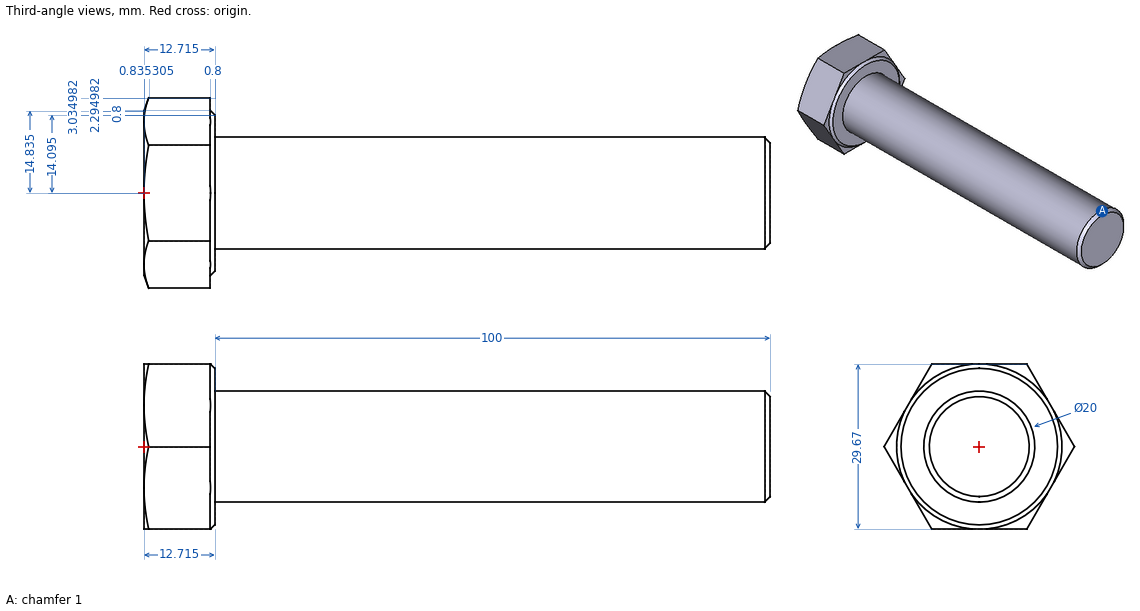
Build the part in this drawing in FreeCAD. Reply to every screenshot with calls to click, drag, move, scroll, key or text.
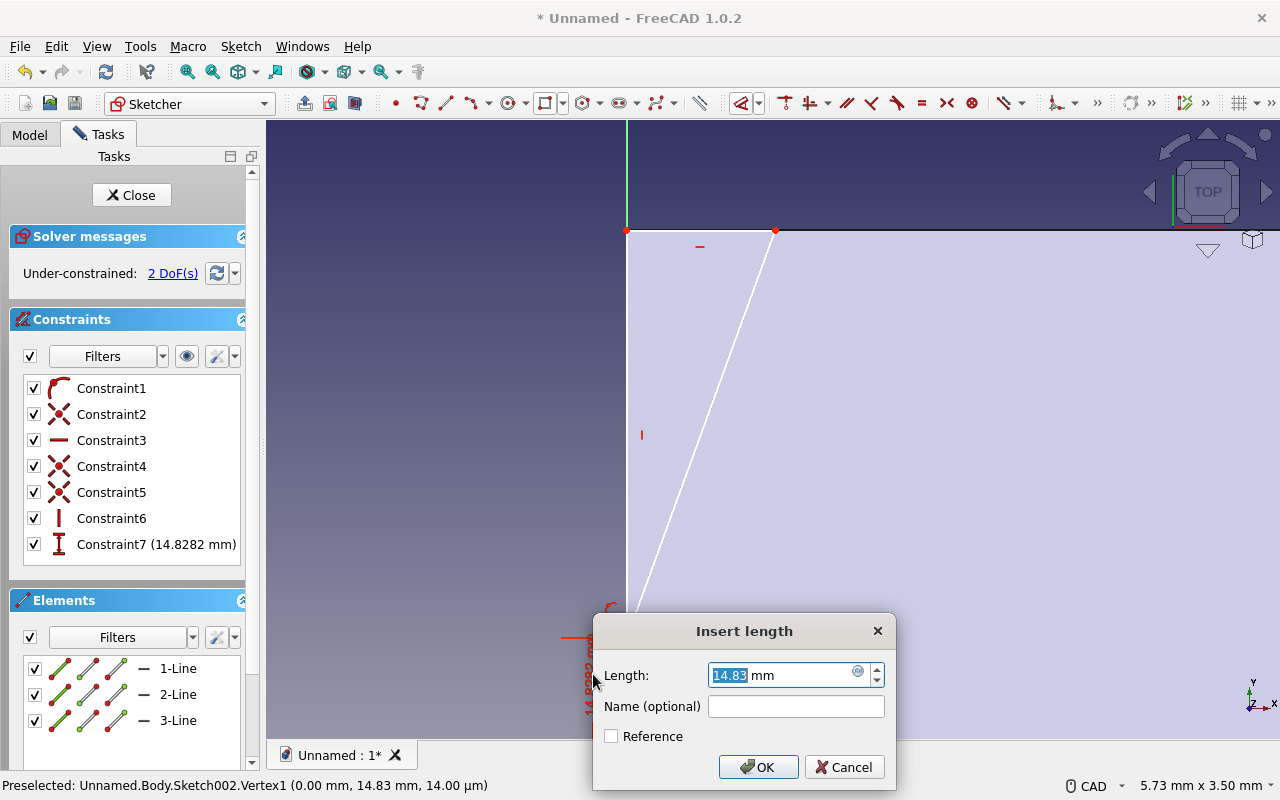
text(14.835)
key(Return)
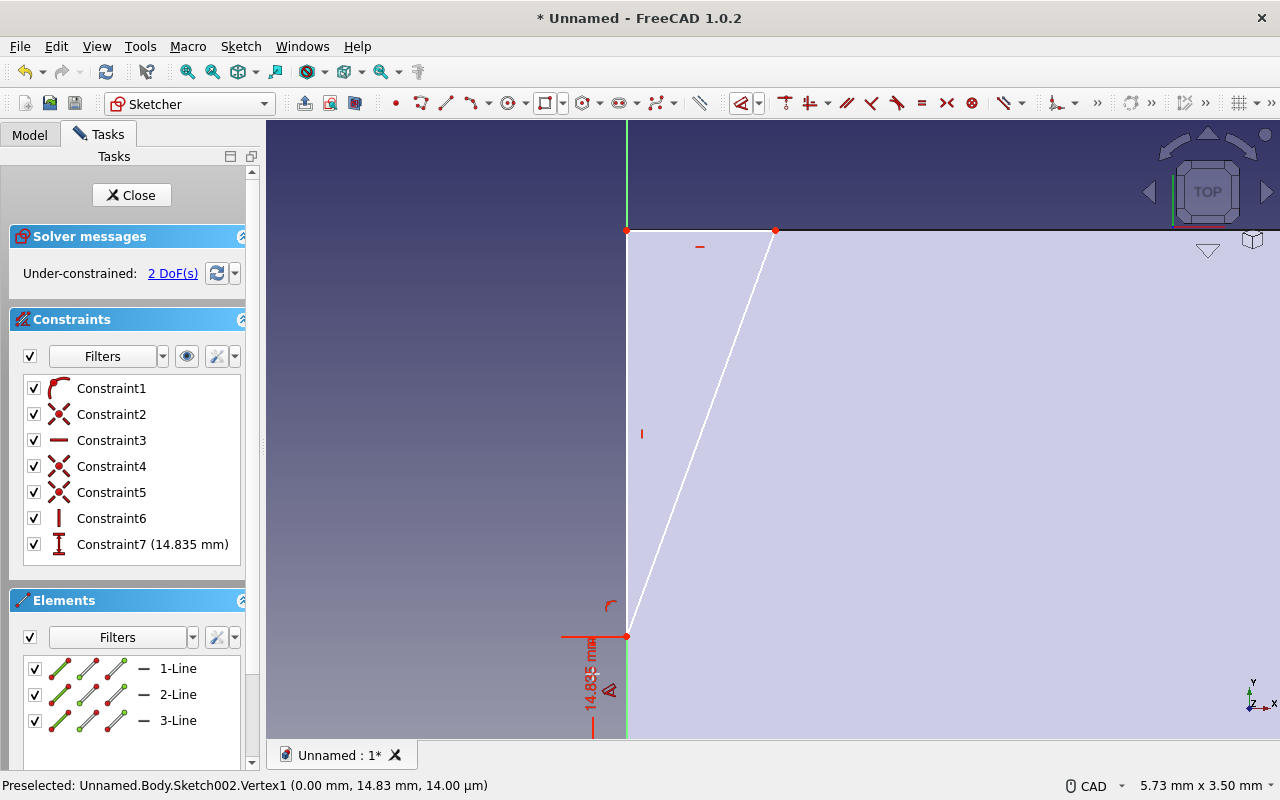
click(731, 231)
click(701, 197)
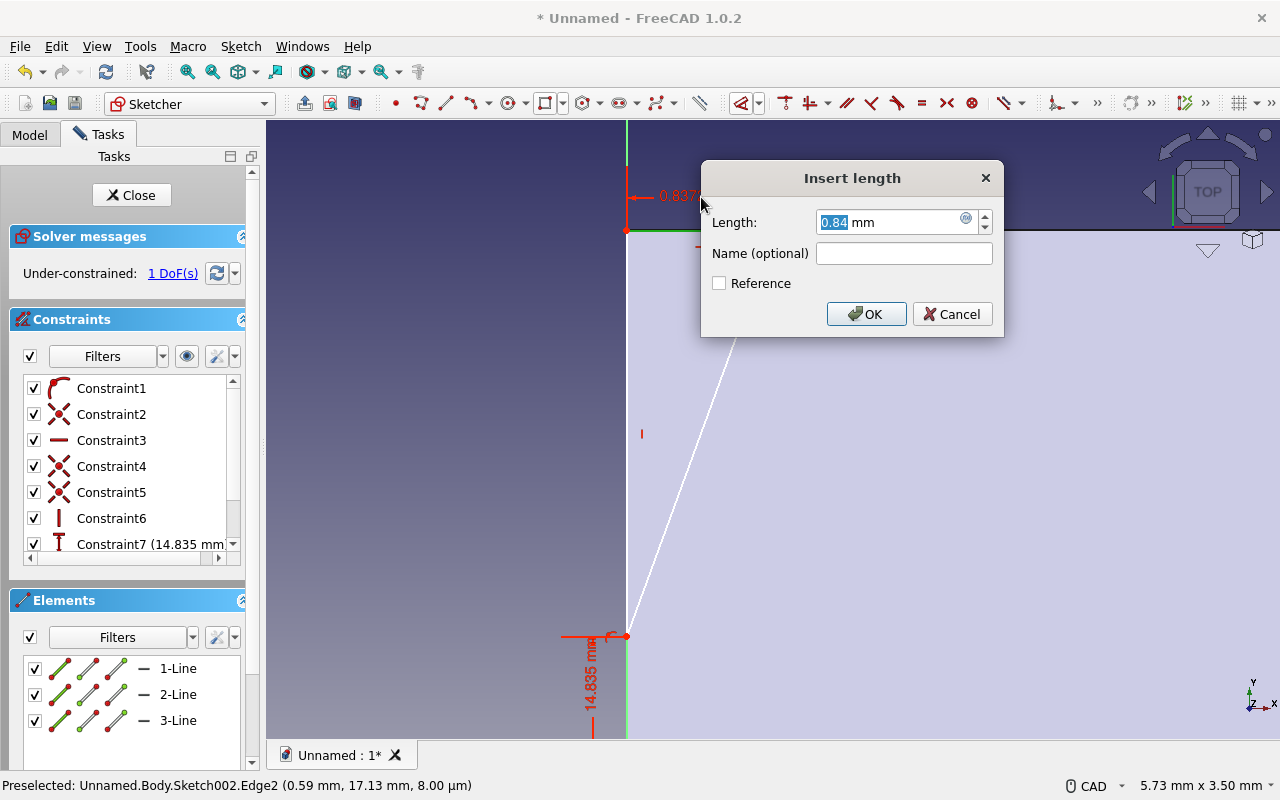
text(0.835305)
key(Return)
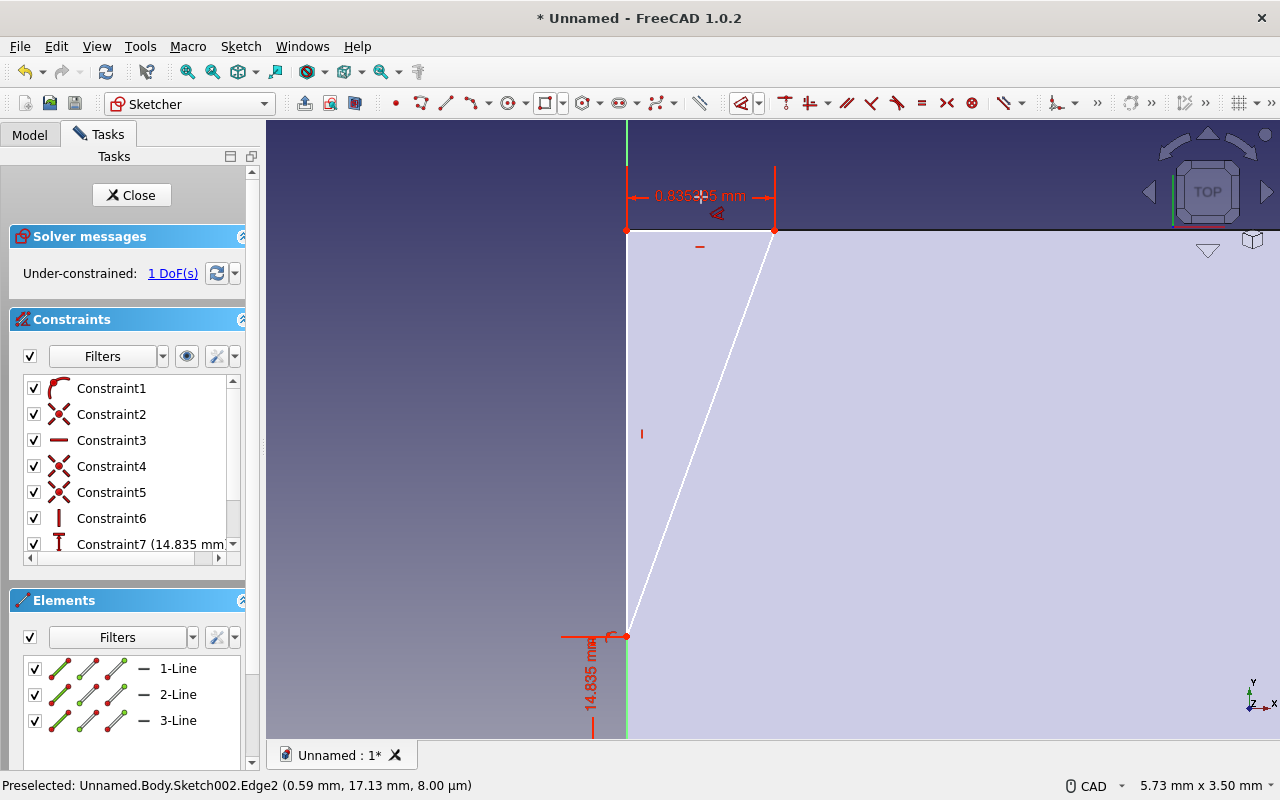
click(627, 353)
click(593, 434)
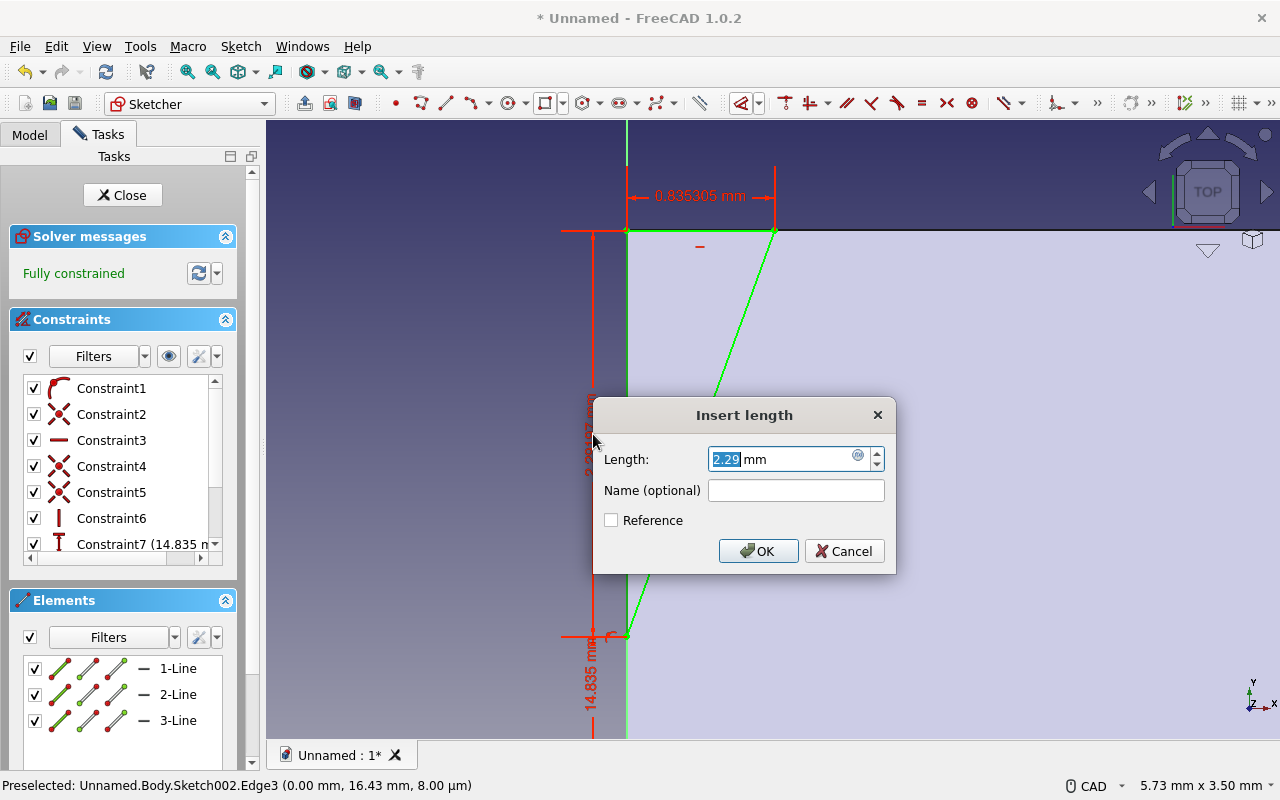
text(2.294982)
key(Return)
key(Escape)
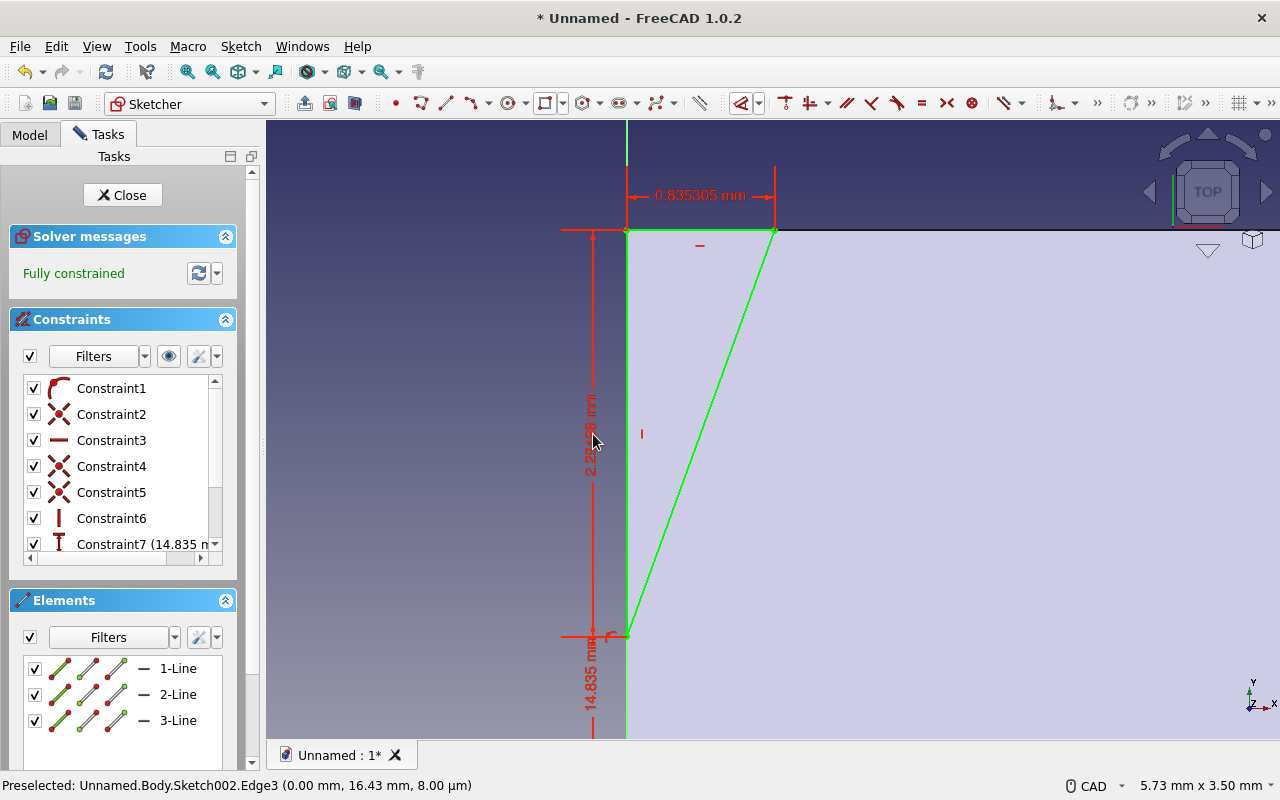
click(123, 195)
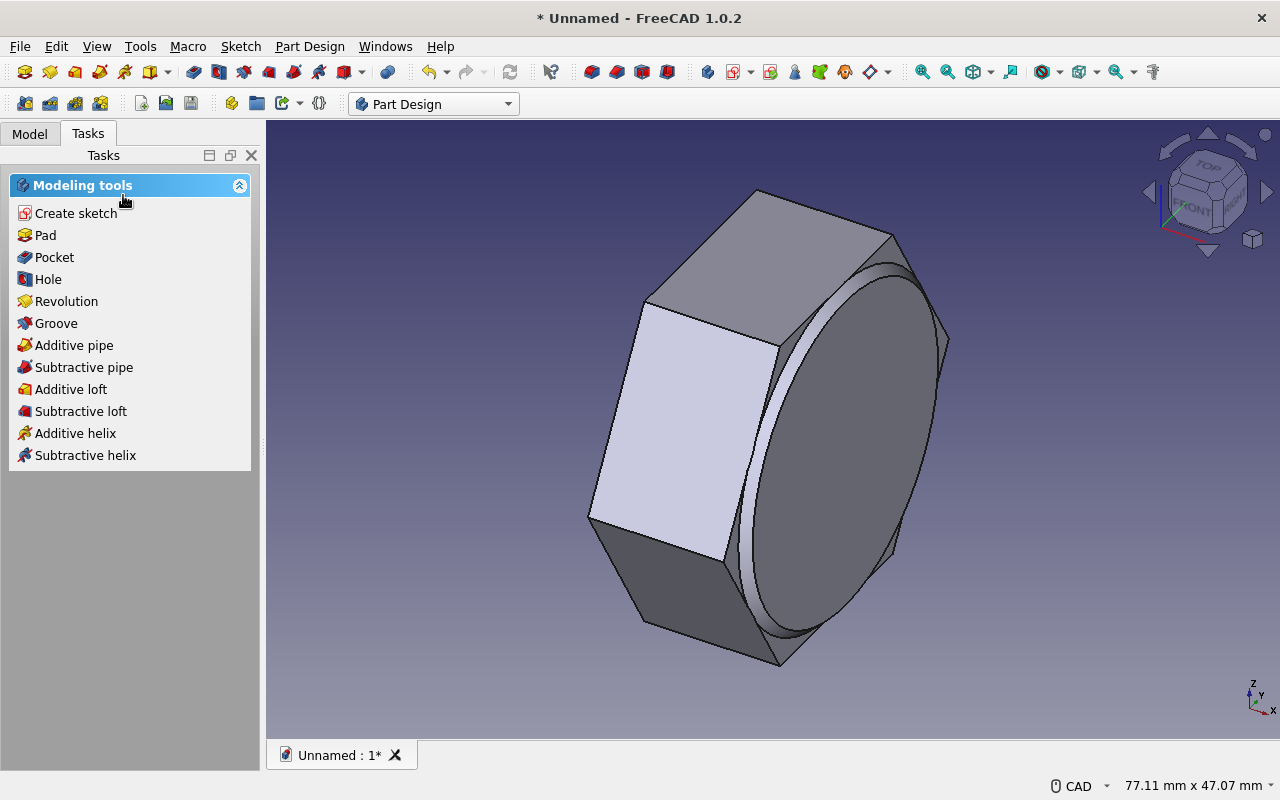
click(244, 72)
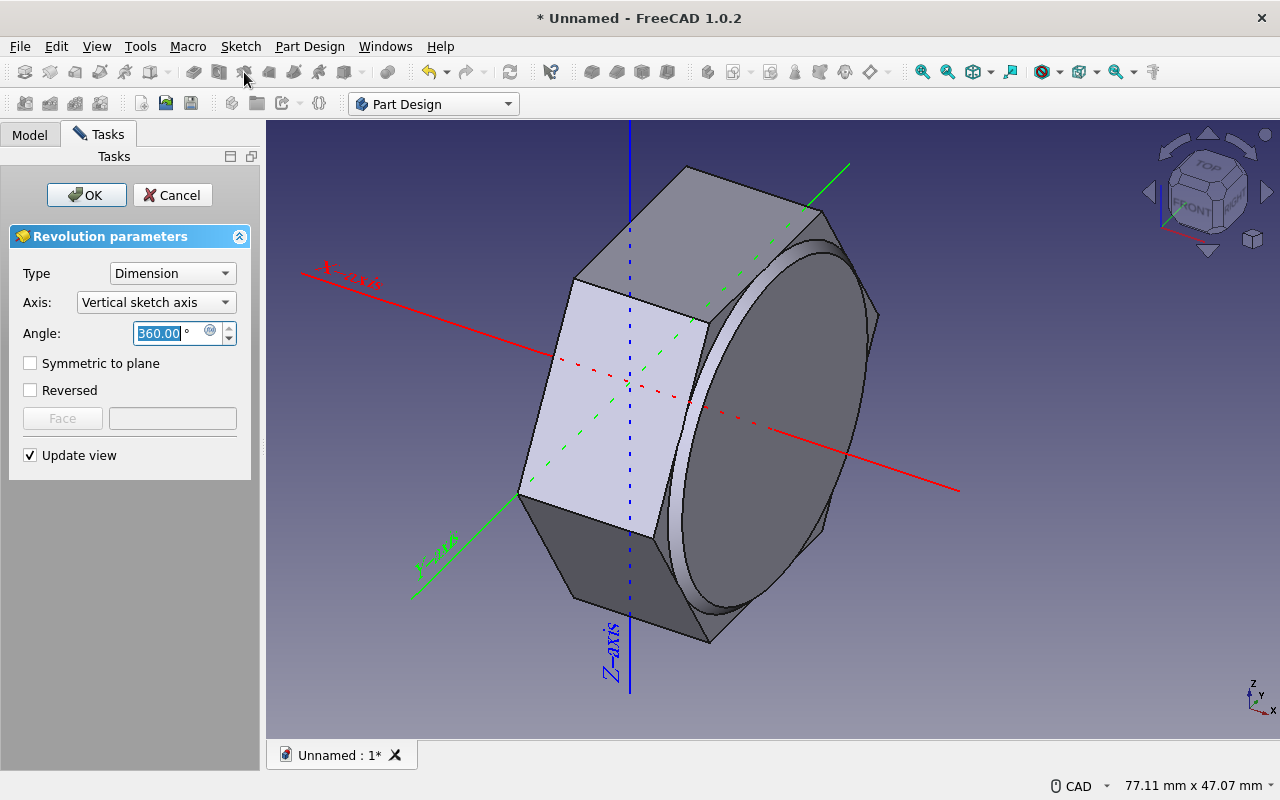
click(157, 302)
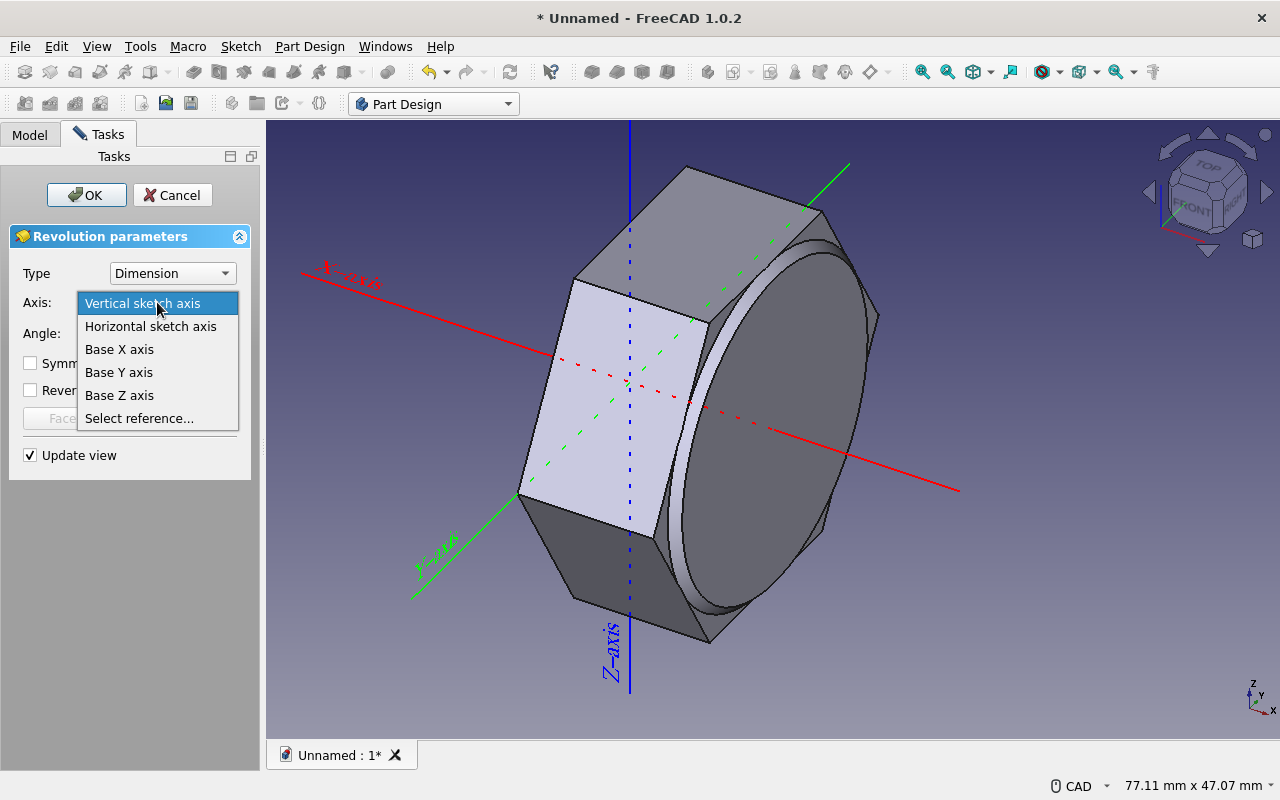
click(156, 326)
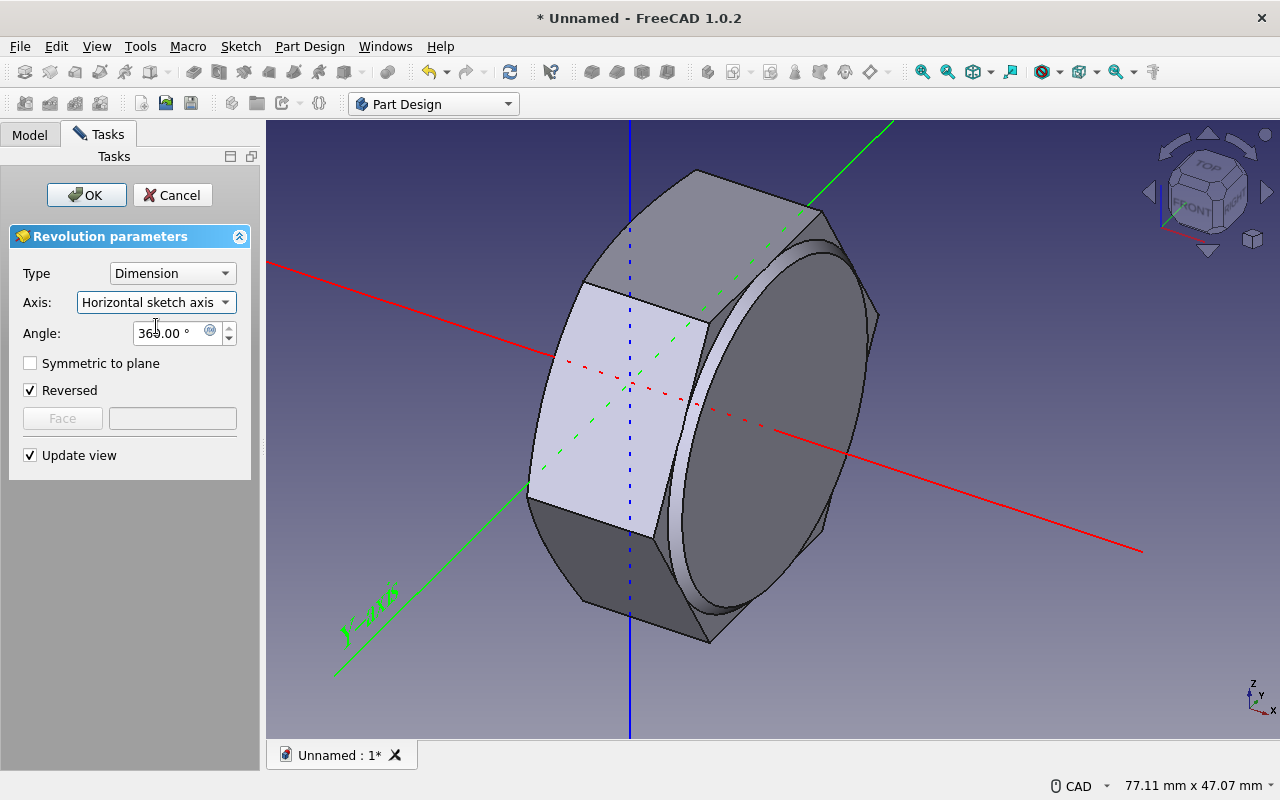
click(87, 195)